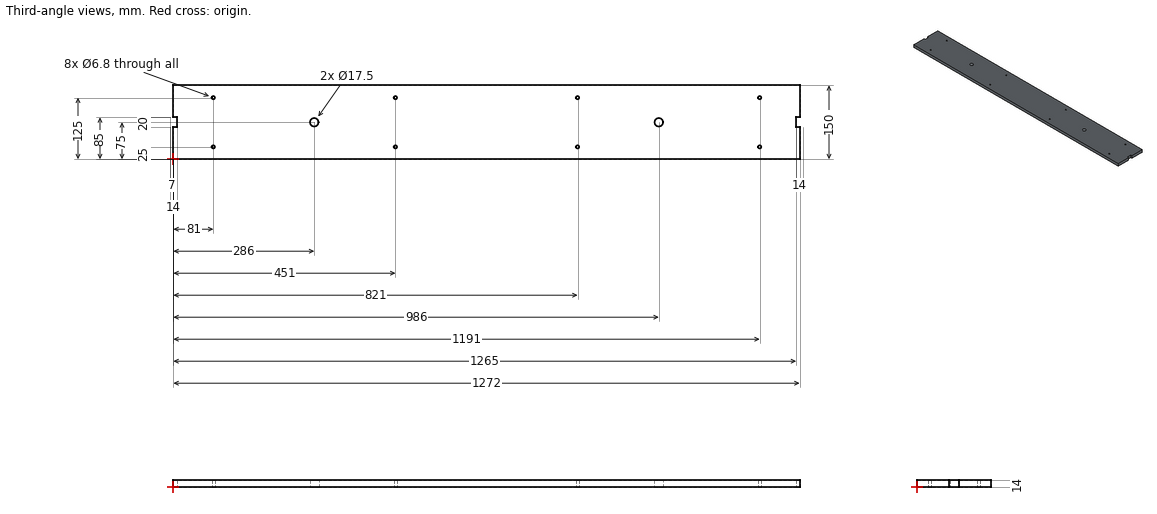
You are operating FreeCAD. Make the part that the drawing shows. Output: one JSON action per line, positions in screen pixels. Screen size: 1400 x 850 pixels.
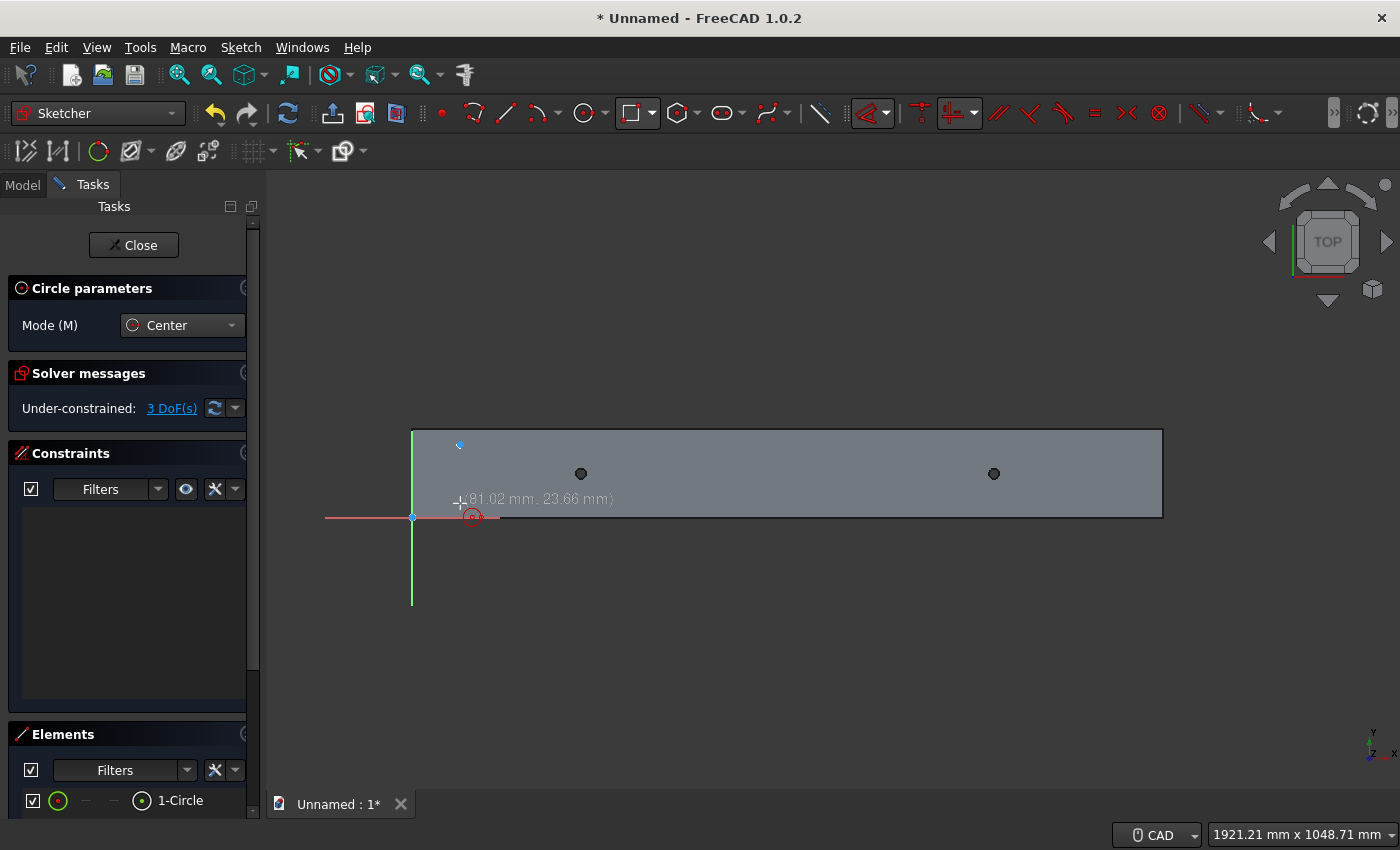
{"action": "left_click", "coordinate": [460, 503]}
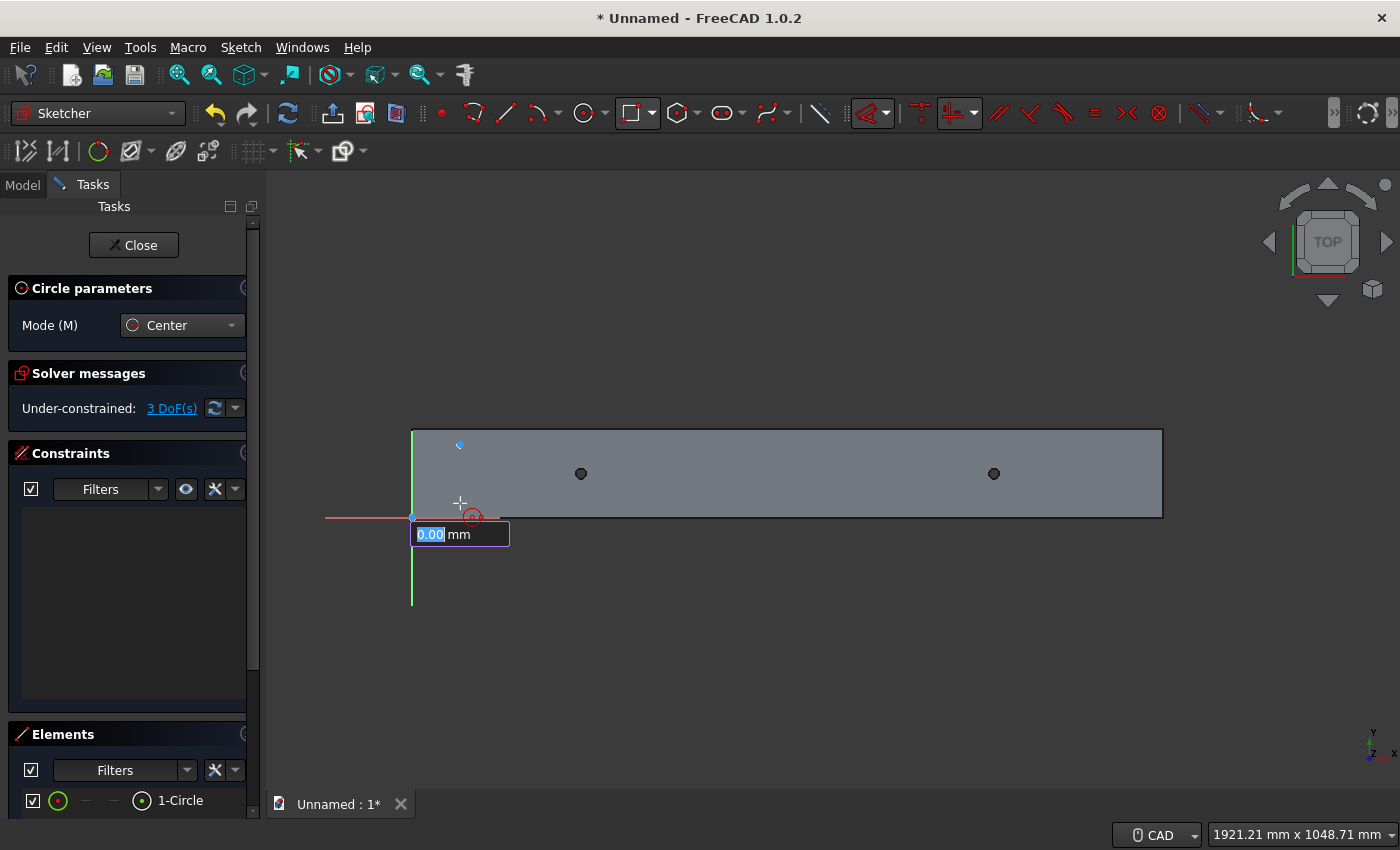
{"action": "scroll", "coordinate": [461, 502], "scroll_direction": "up", "scroll_amount": 11}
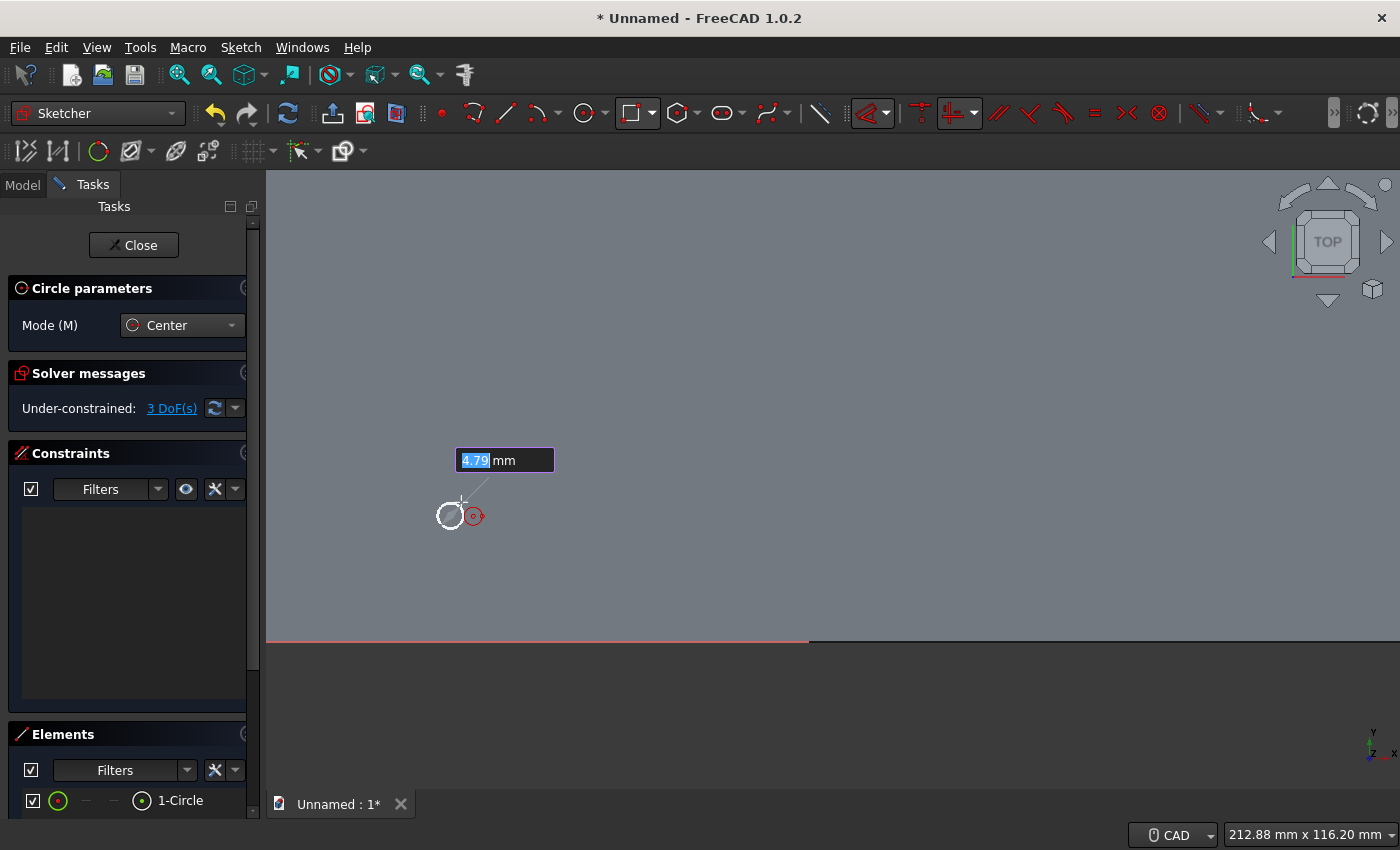
{"action": "left_click", "coordinate": [463, 496]}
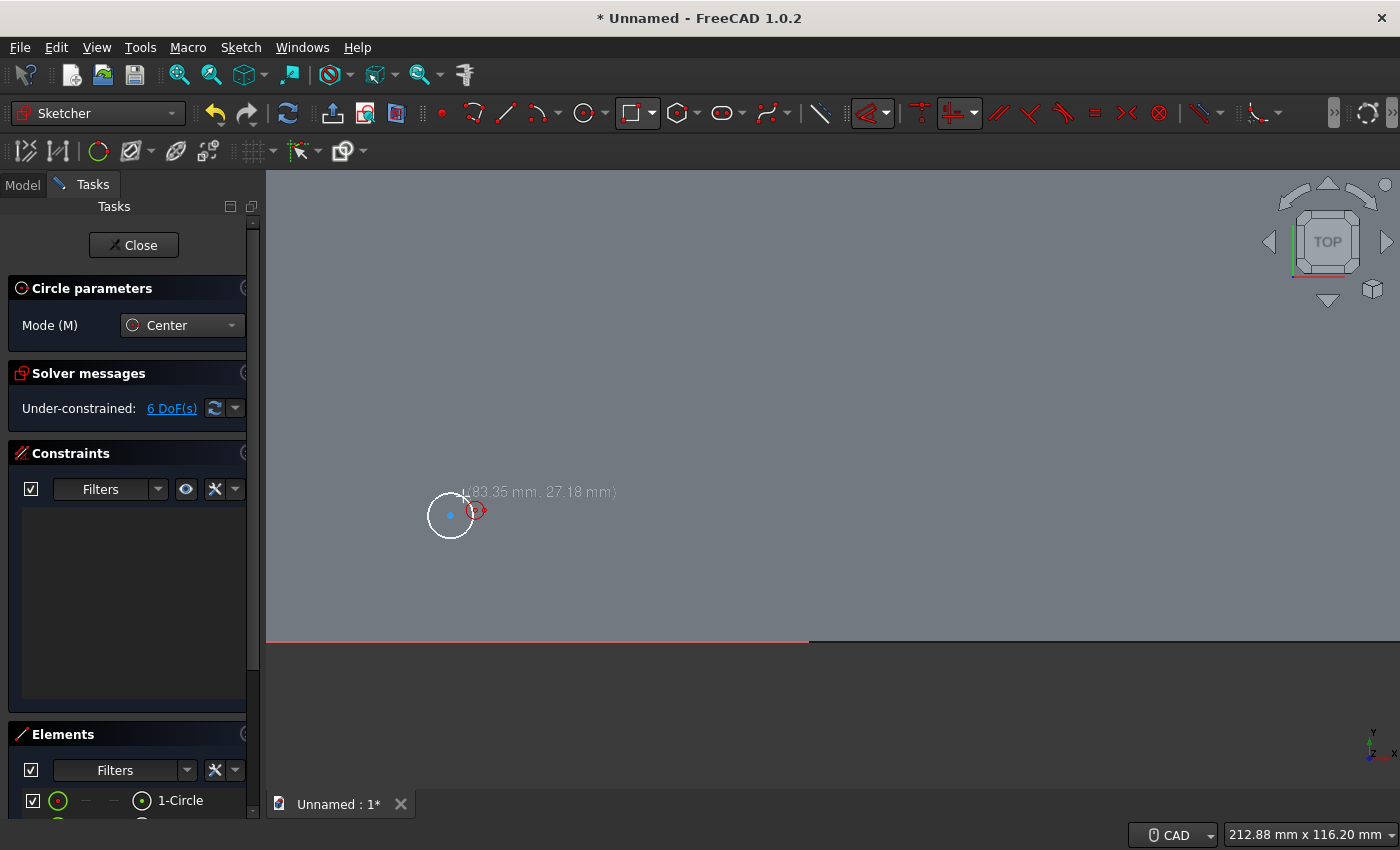
{"action": "scroll", "coordinate": [461, 502], "scroll_direction": "down", "scroll_amount": 11}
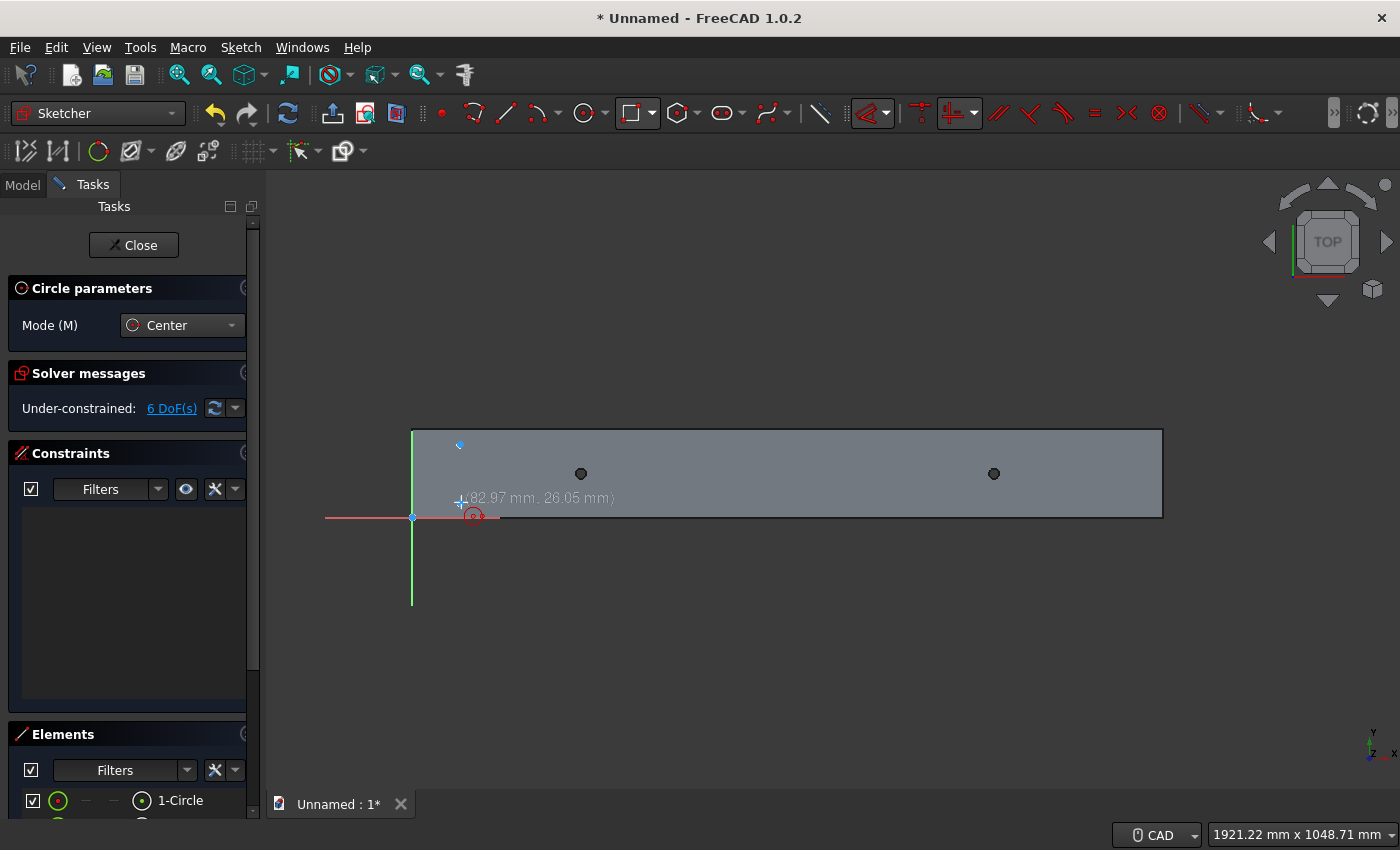
{"action": "scroll", "coordinate": [678, 444], "scroll_direction": "up", "scroll_amount": 13}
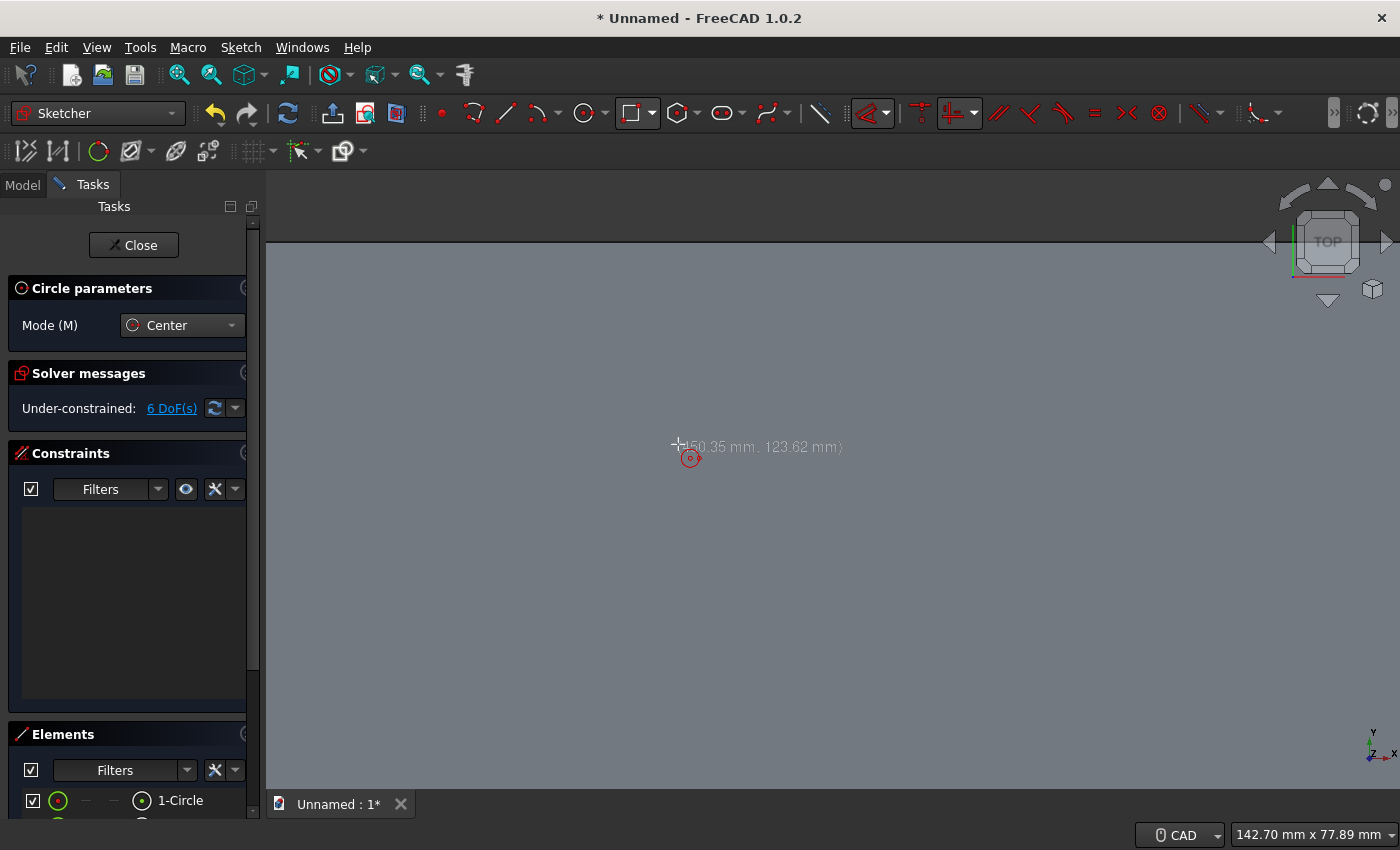
{"action": "scroll", "coordinate": [678, 444], "scroll_direction": "down", "scroll_amount": 13}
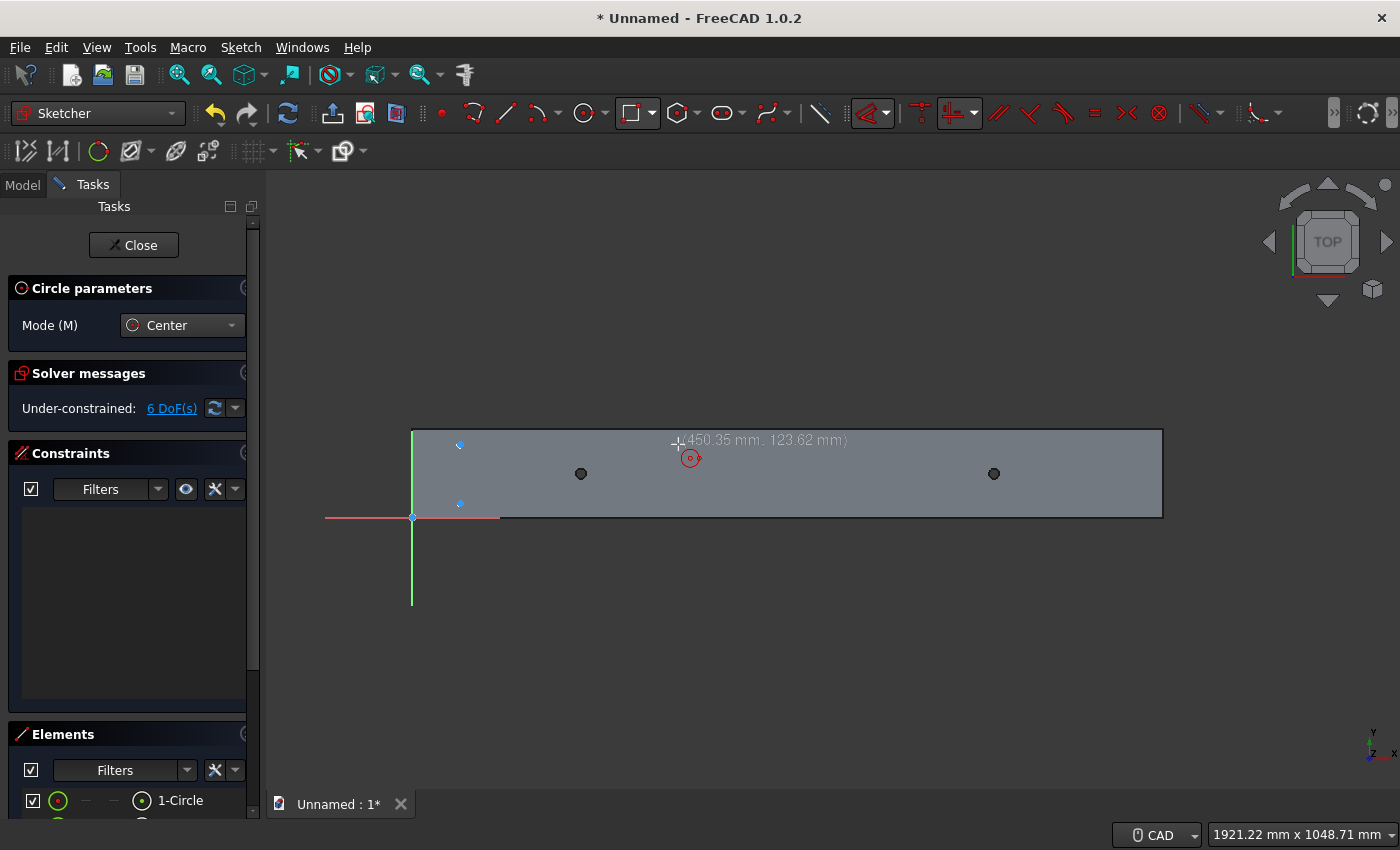
{"action": "left_click", "coordinate": [678, 444]}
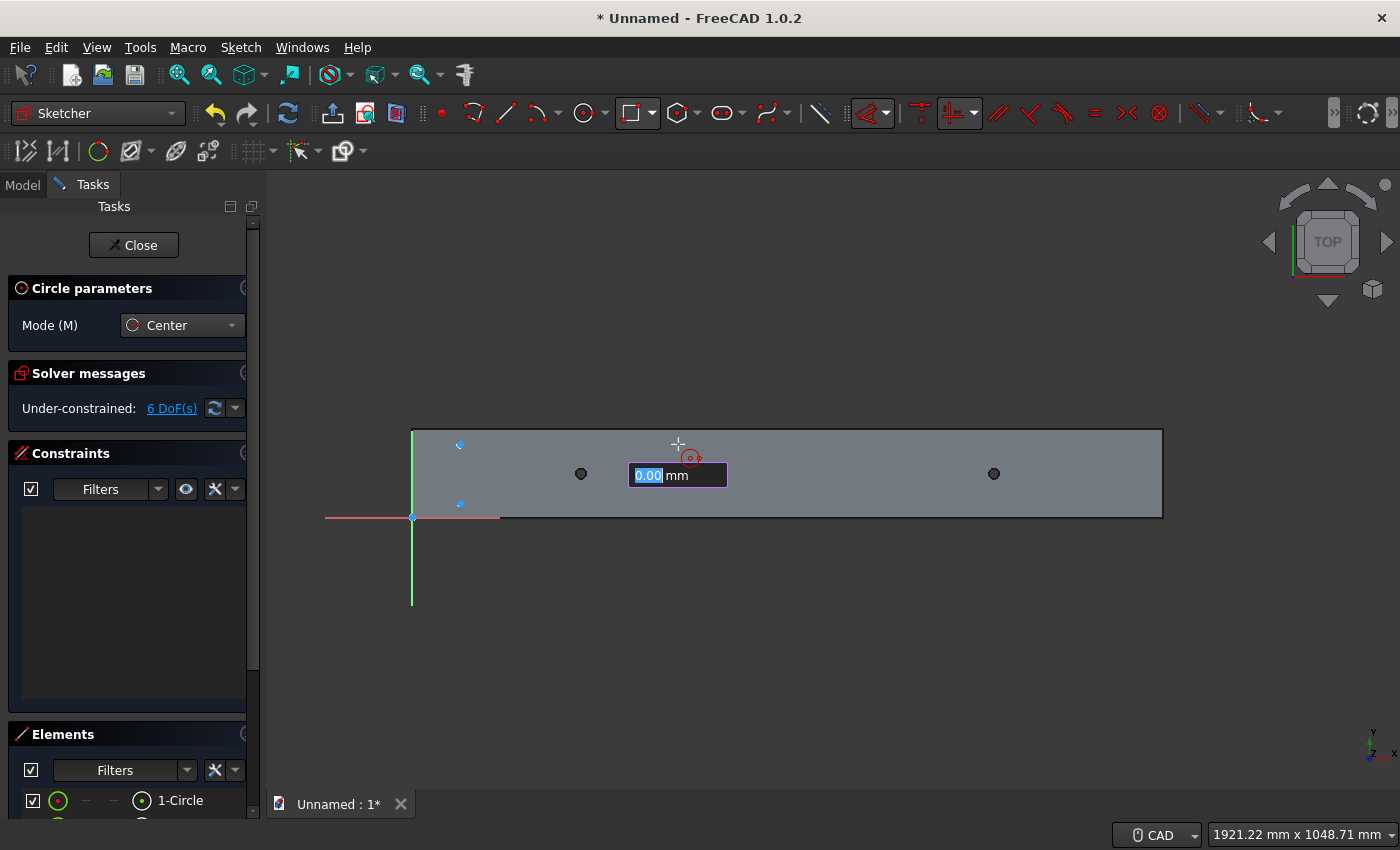
{"action": "scroll", "coordinate": [680, 443], "scroll_direction": "up", "scroll_amount": 11}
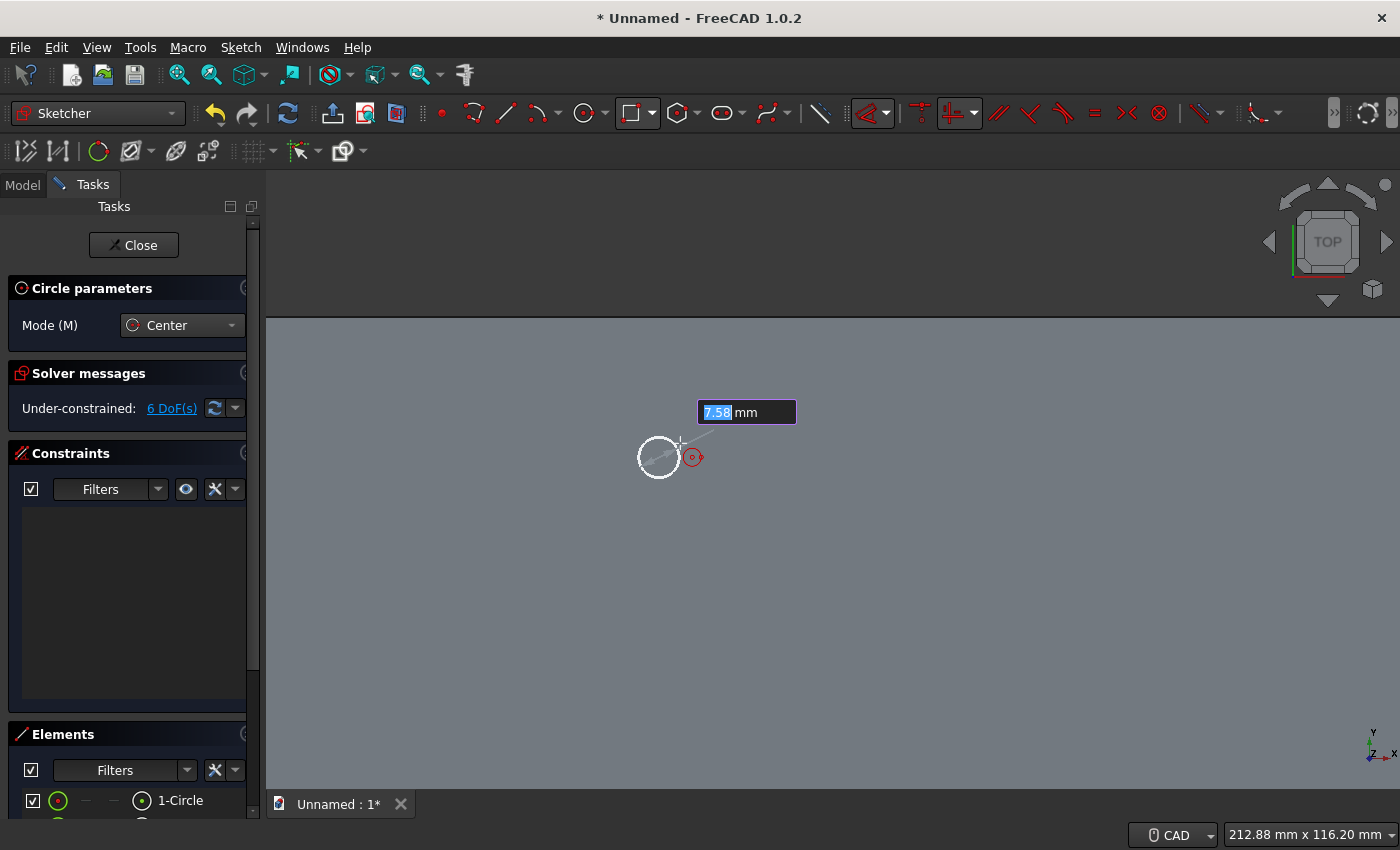
{"action": "left_click", "coordinate": [675, 437]}